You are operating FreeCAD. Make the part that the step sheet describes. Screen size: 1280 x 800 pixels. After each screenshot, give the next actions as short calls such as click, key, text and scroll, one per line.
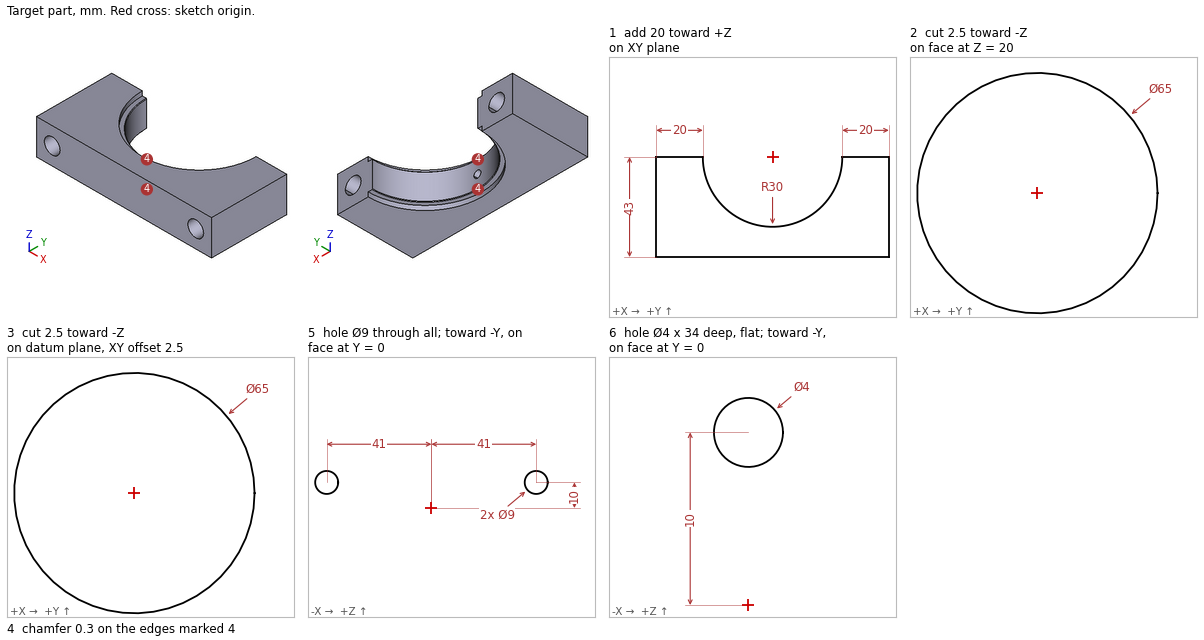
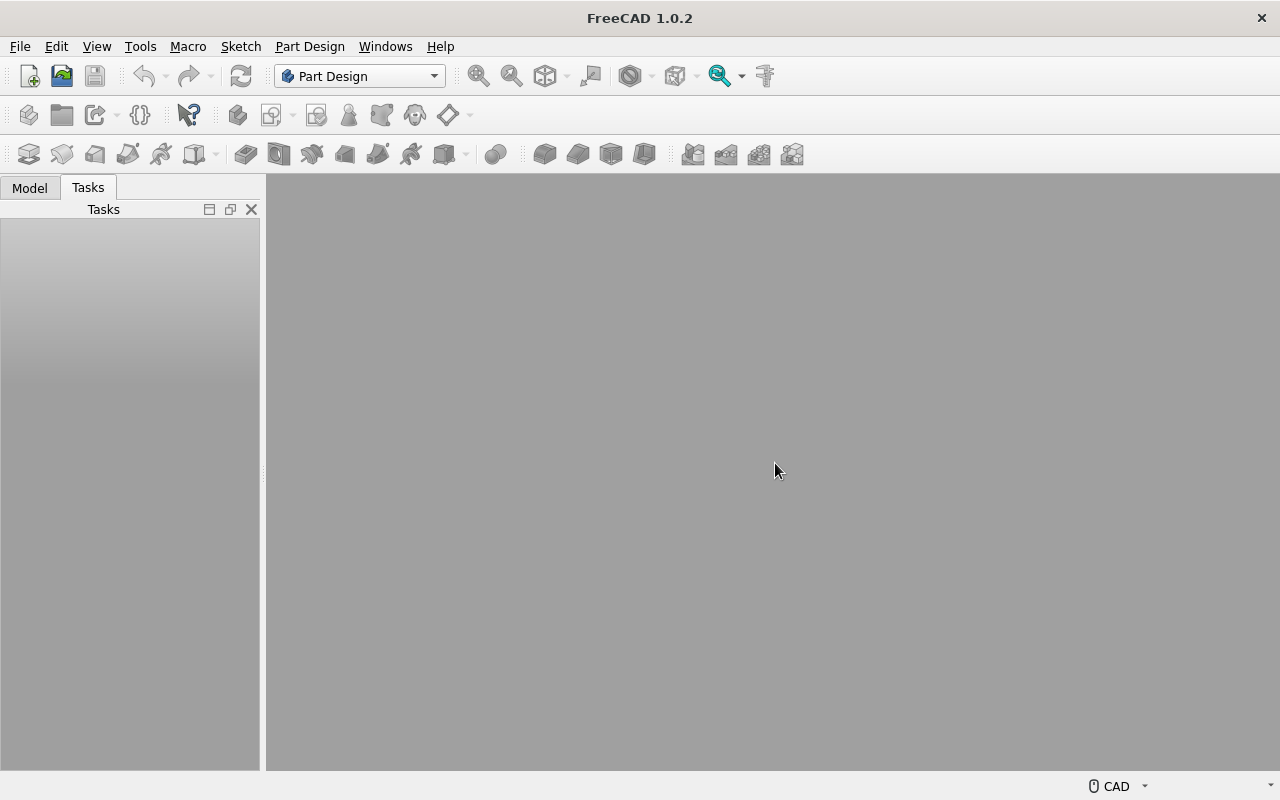
key(ctrl+n)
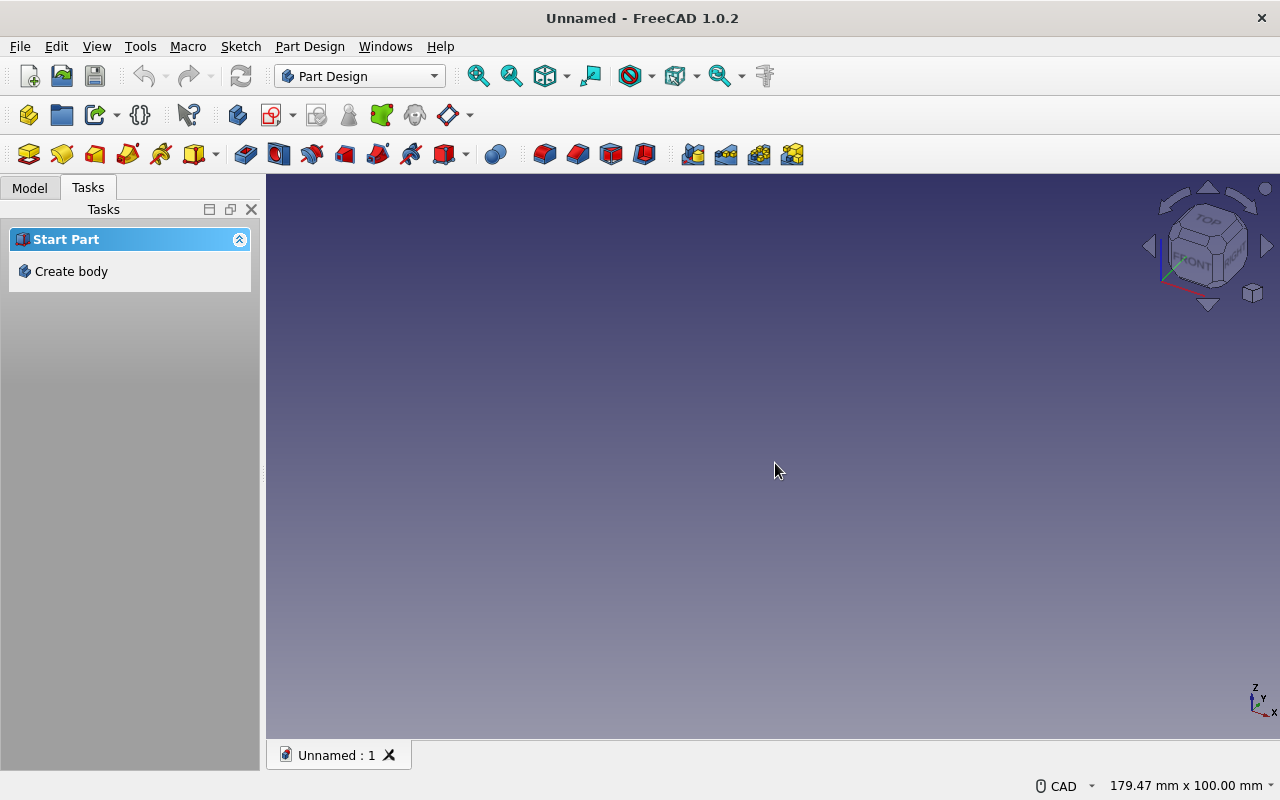
click(270, 116)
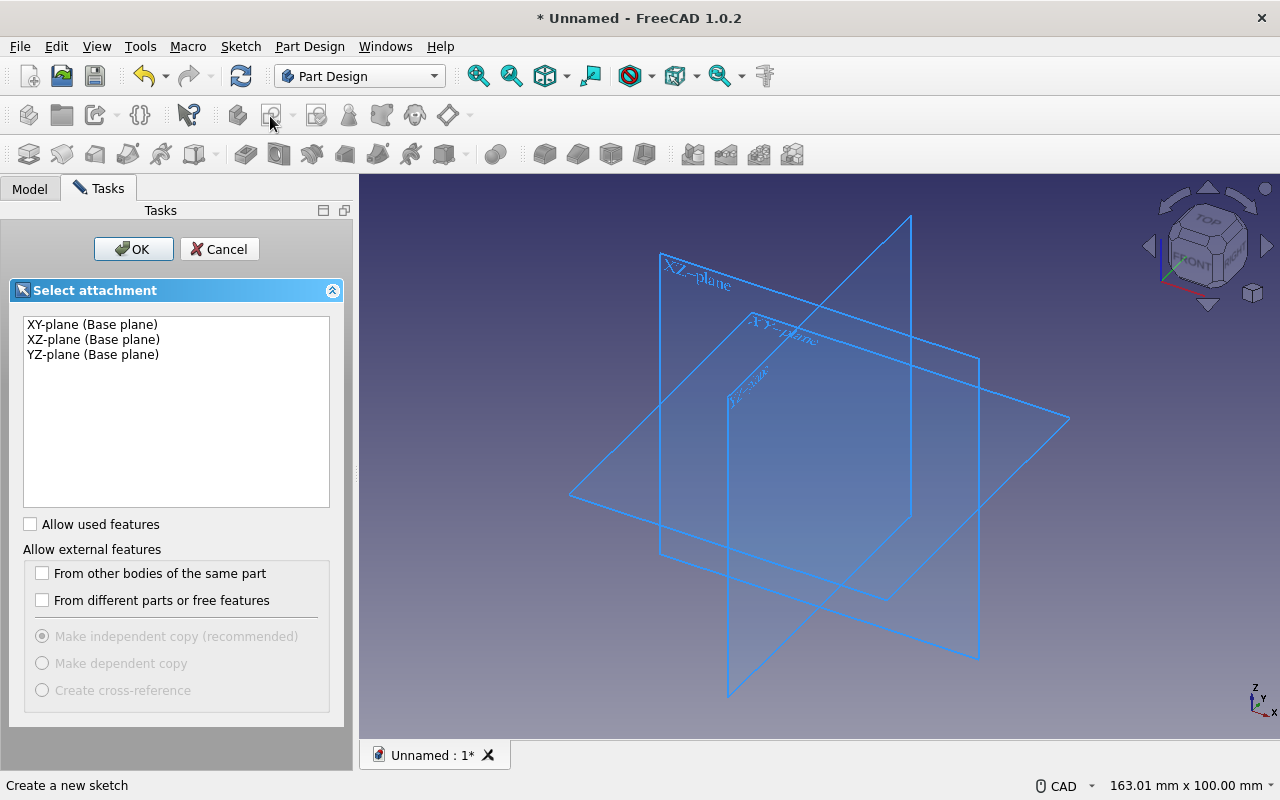
click(84, 324)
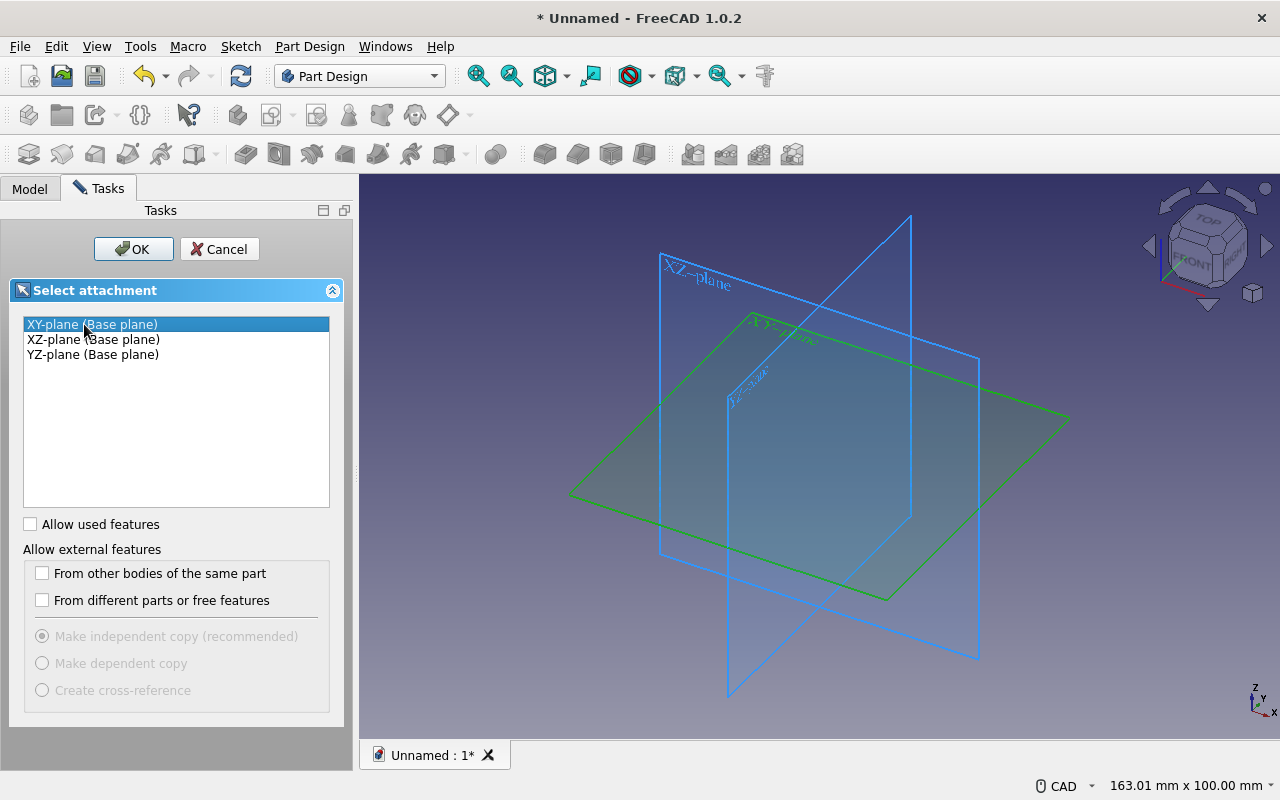
click(134, 249)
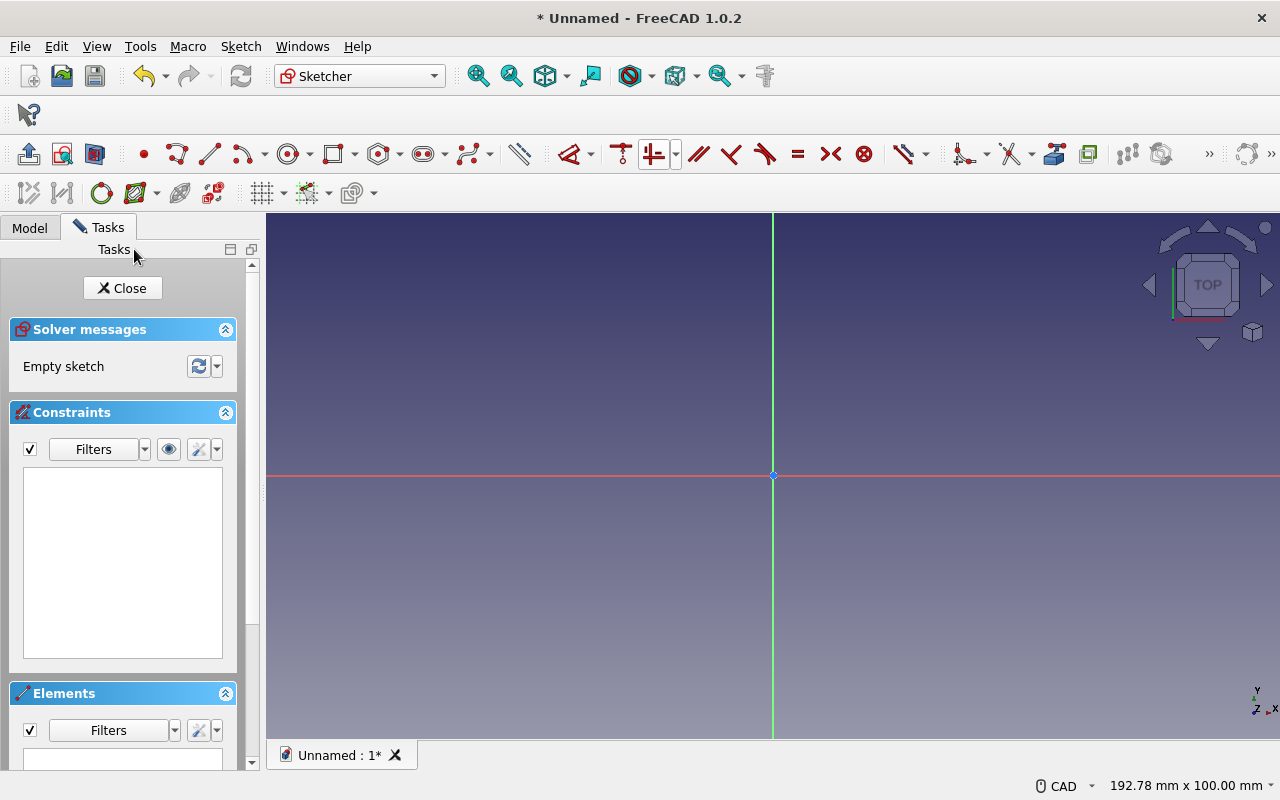
scroll(395, 241, down, 1)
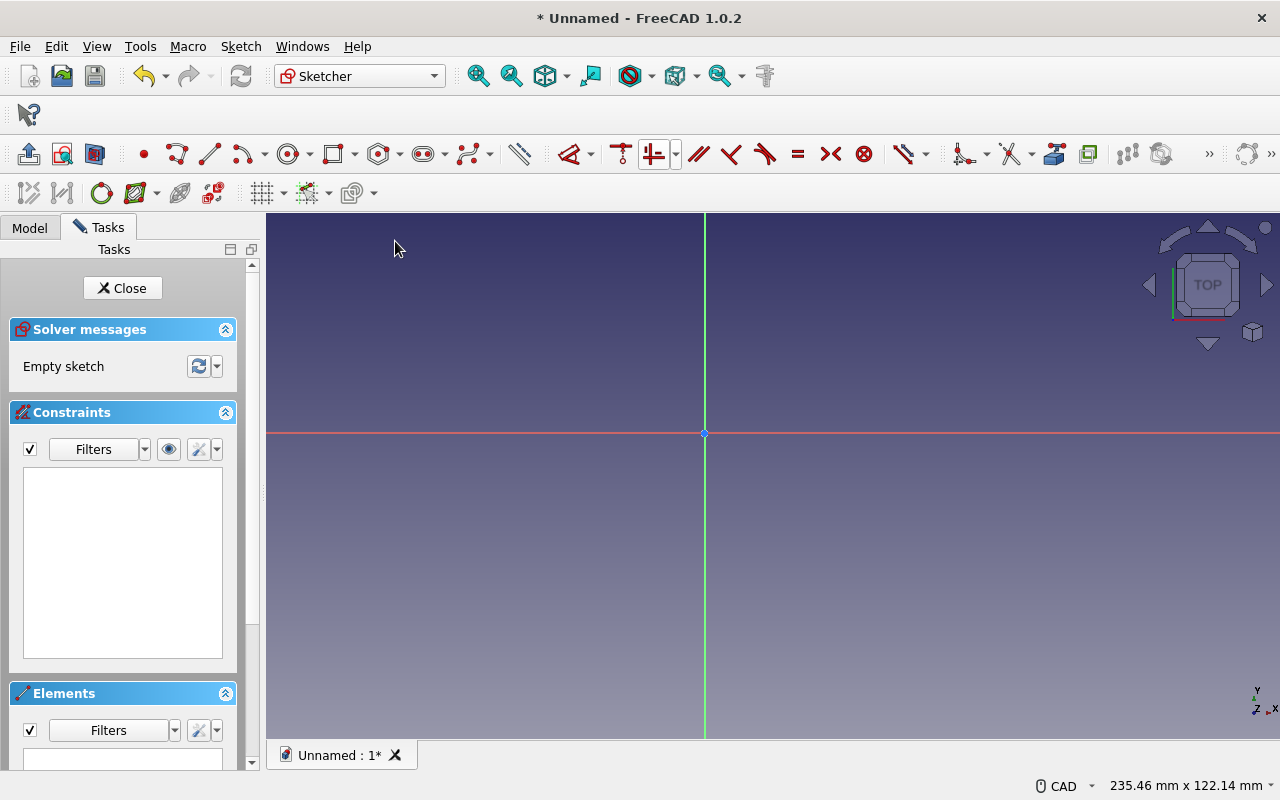
click(177, 154)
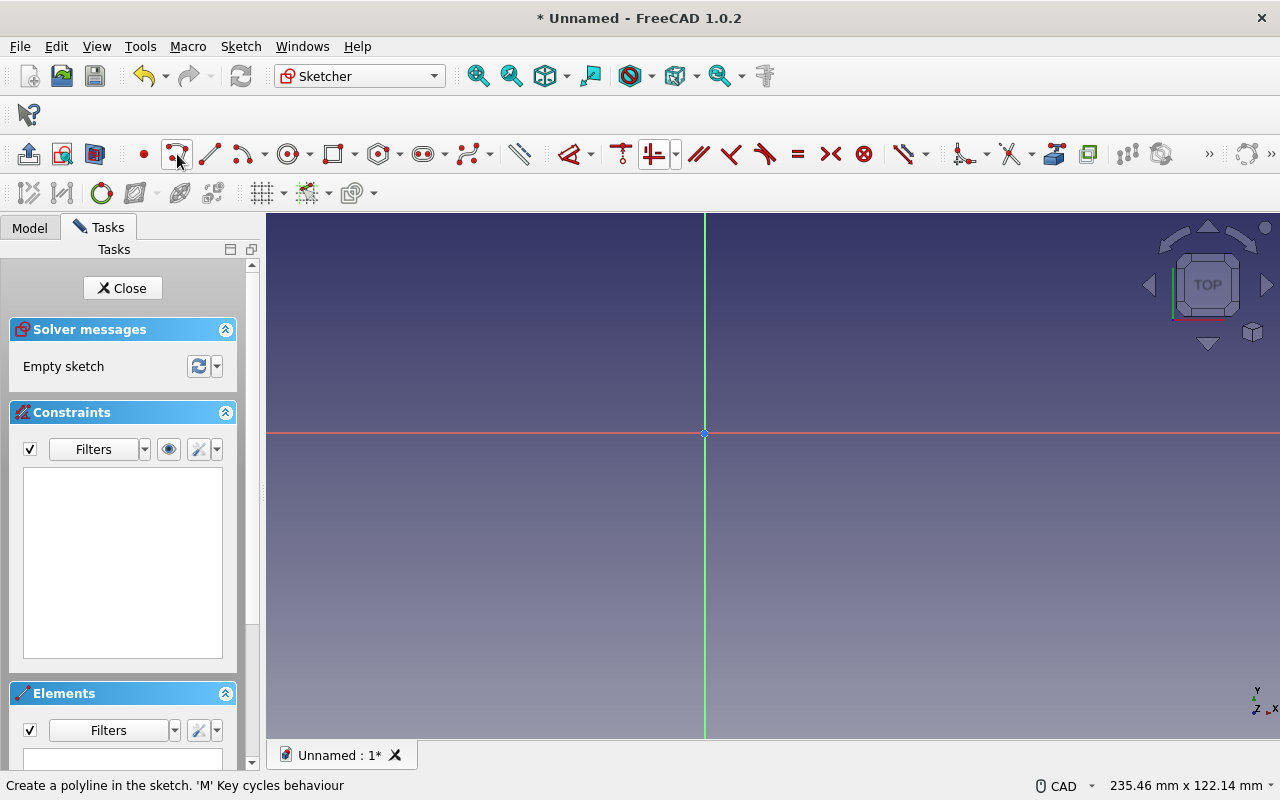
click(575, 433)
click(489, 442)
click(489, 619)
click(920, 619)
click(920, 433)
click(834, 442)
right_click(834, 442)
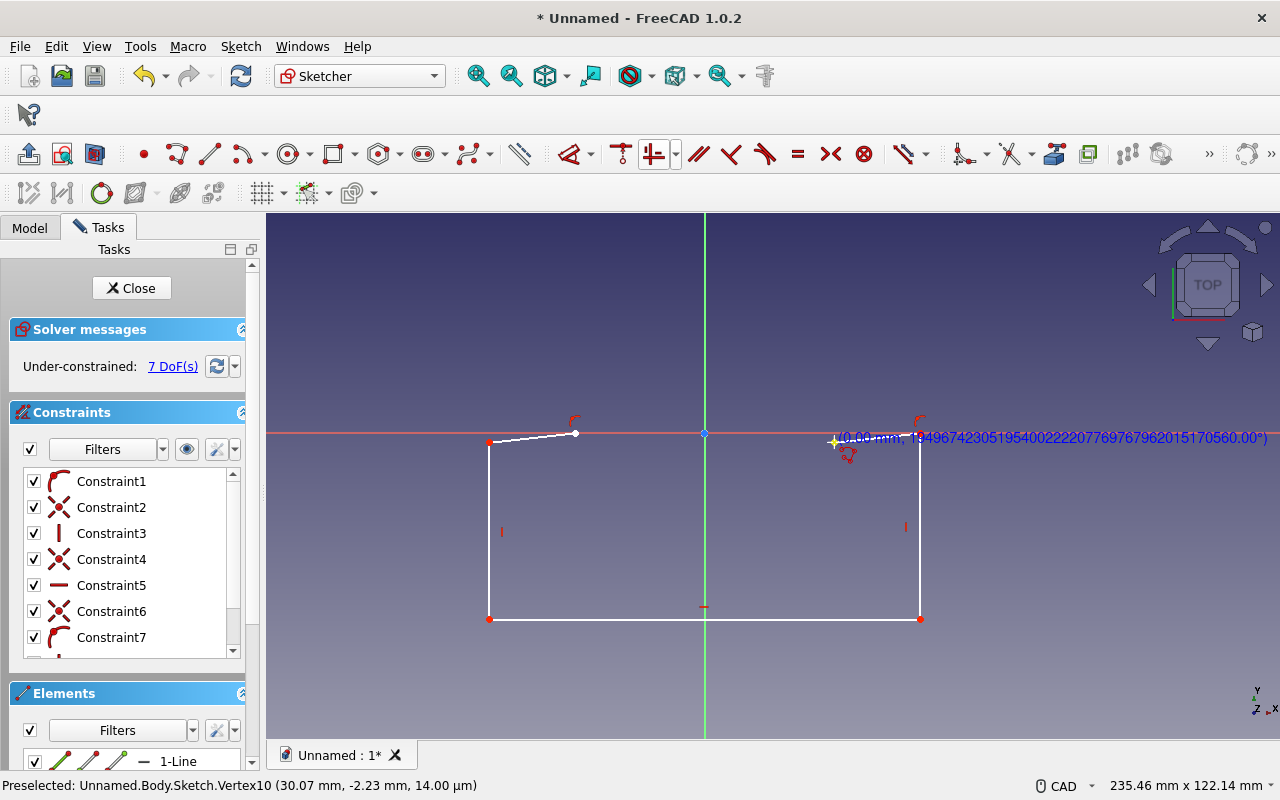
key(g)
key(3)
key(a)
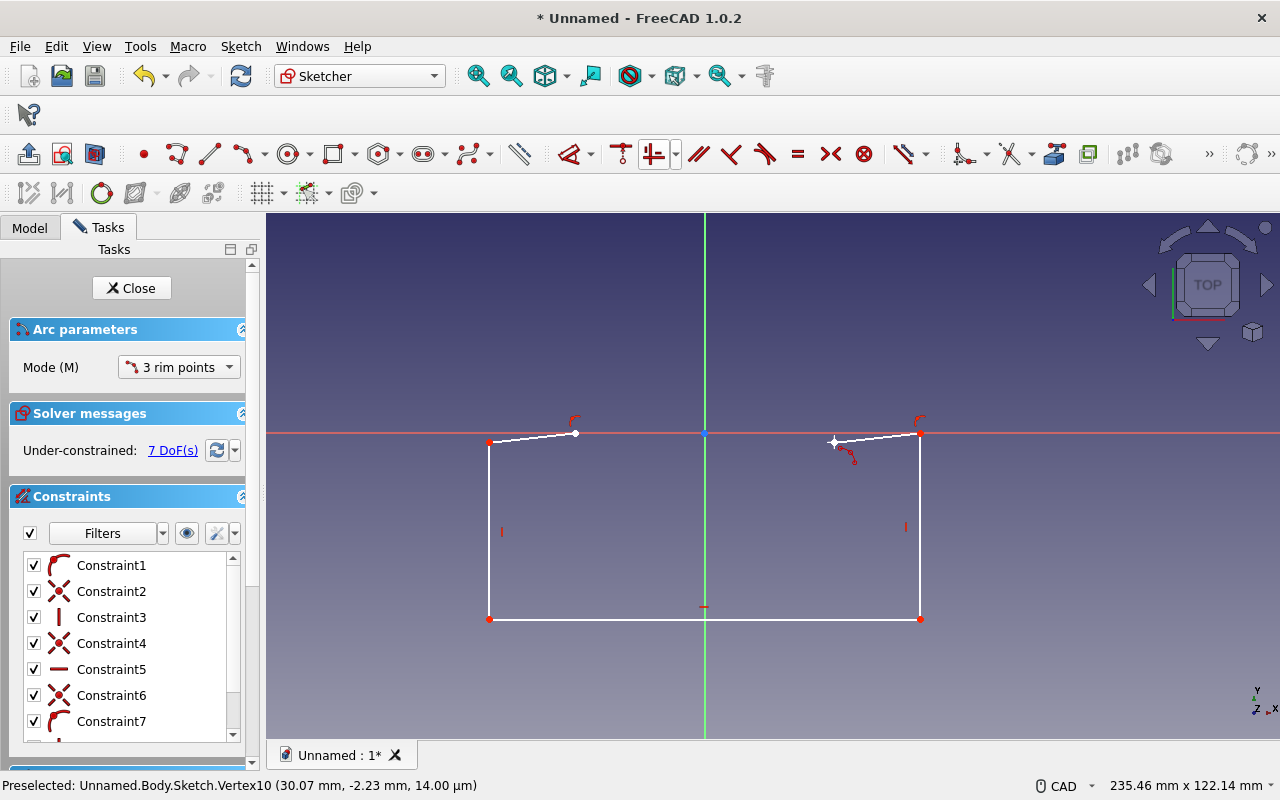
click(834, 443)
click(575, 433)
click(665, 556)
key(Escape)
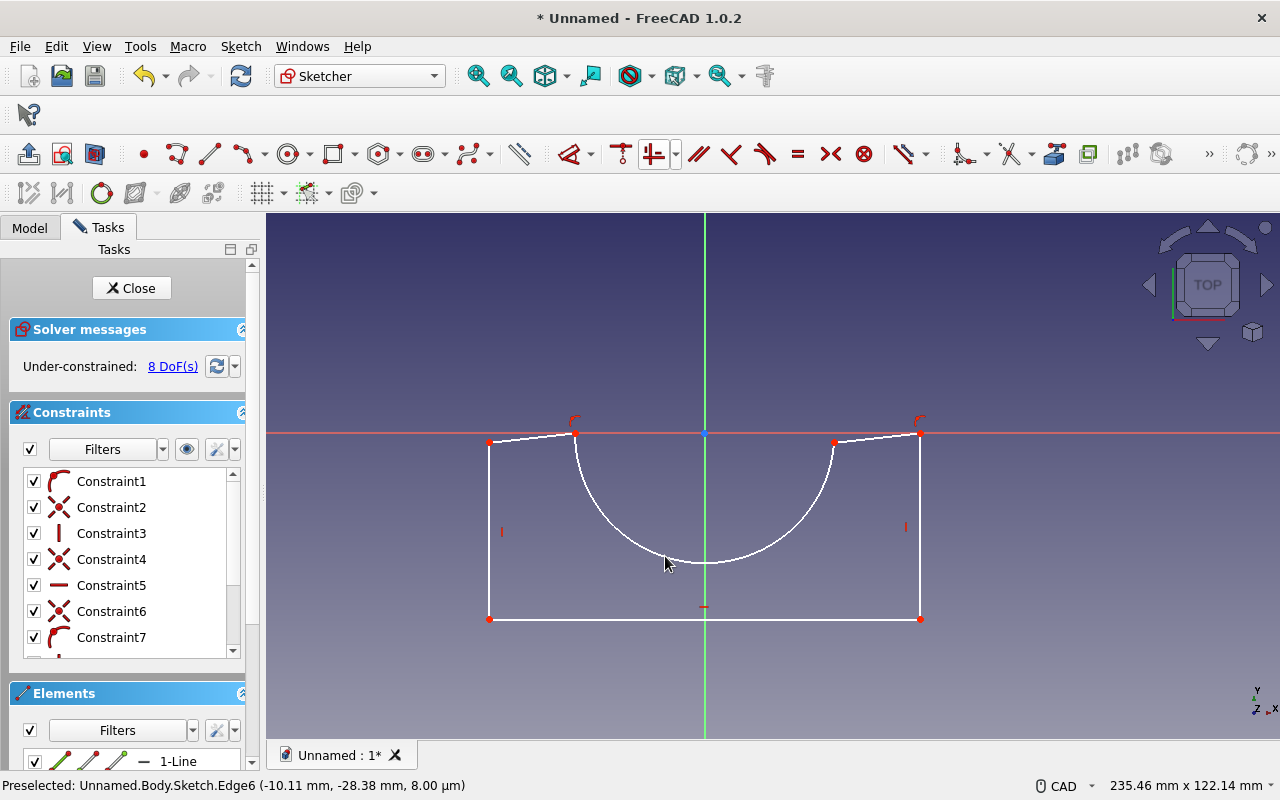
click(549, 436)